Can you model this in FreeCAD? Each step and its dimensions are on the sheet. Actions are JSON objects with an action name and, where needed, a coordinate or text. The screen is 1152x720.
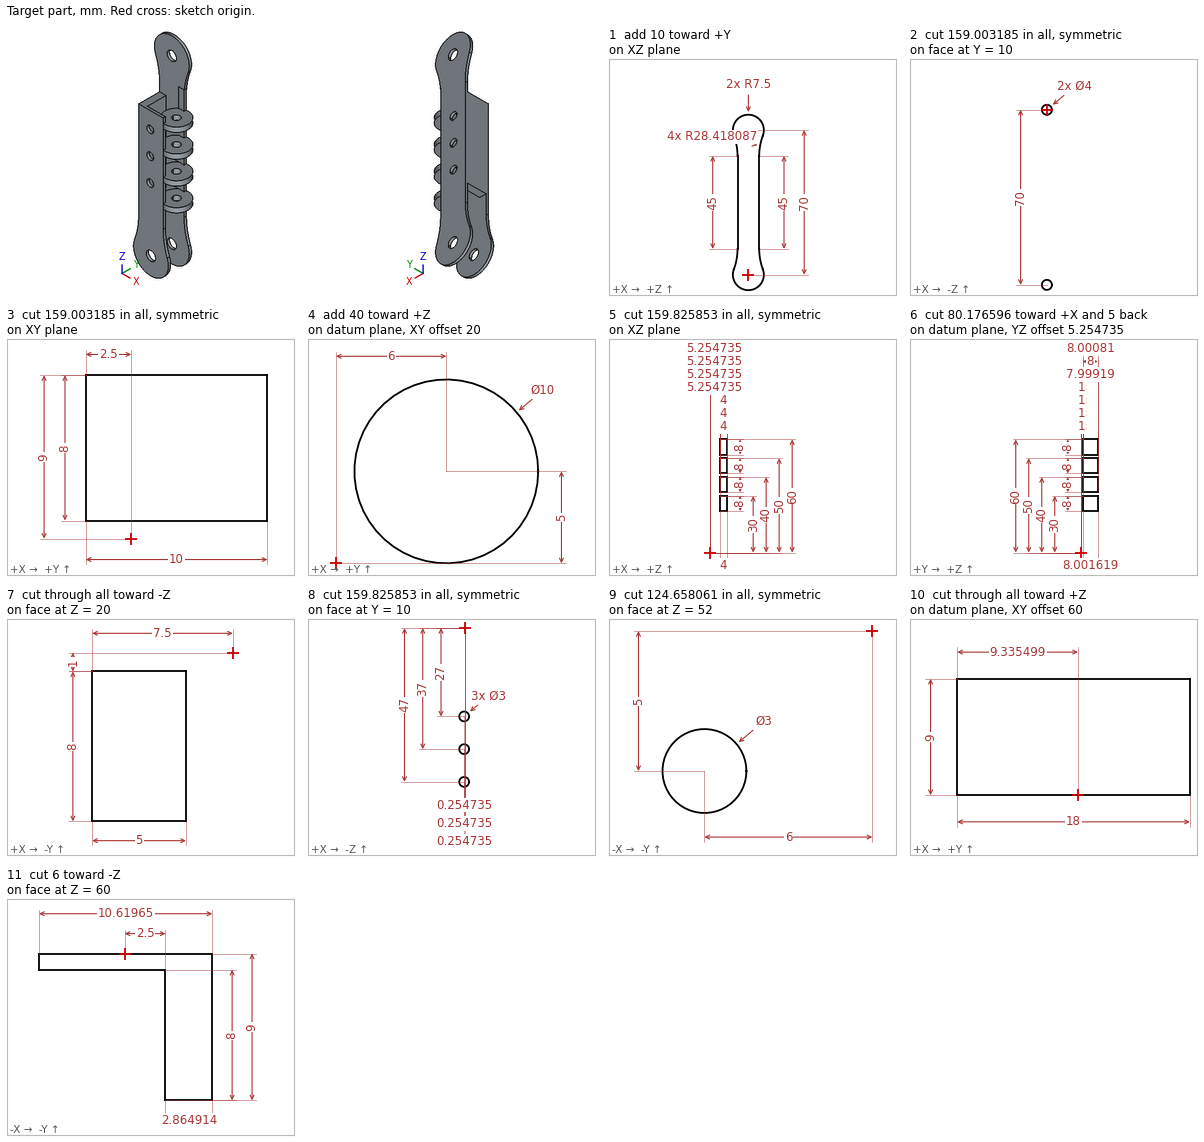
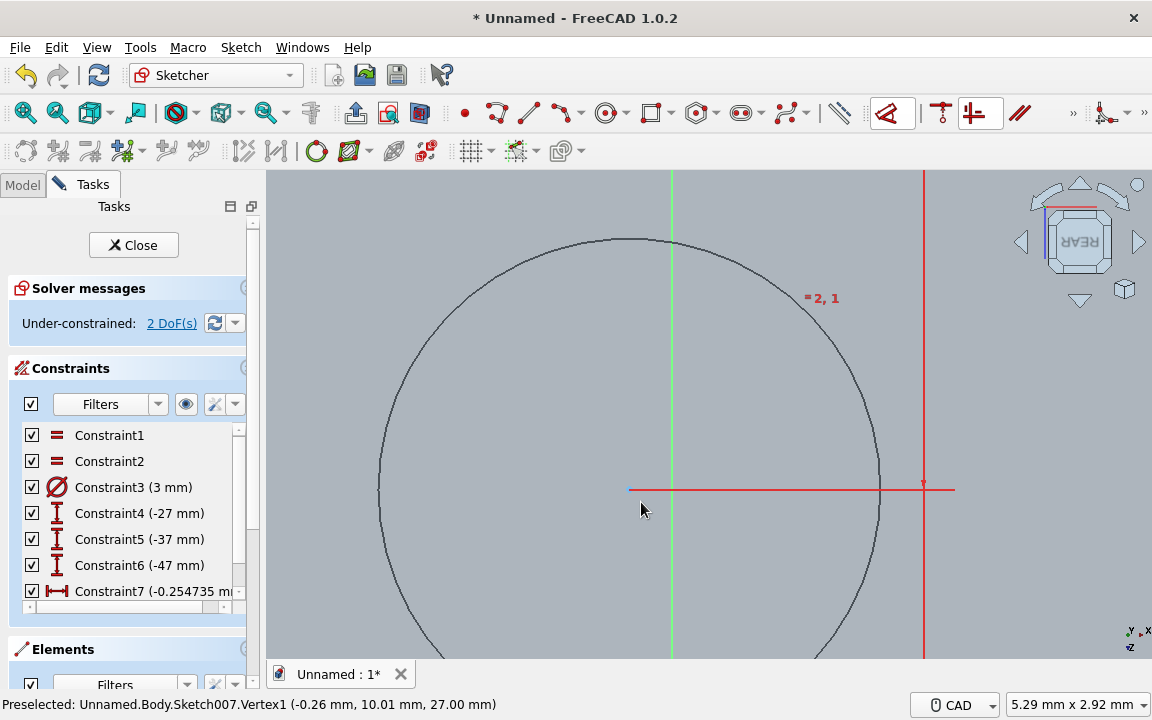
{"action": "left_click", "coordinate": [629, 490]}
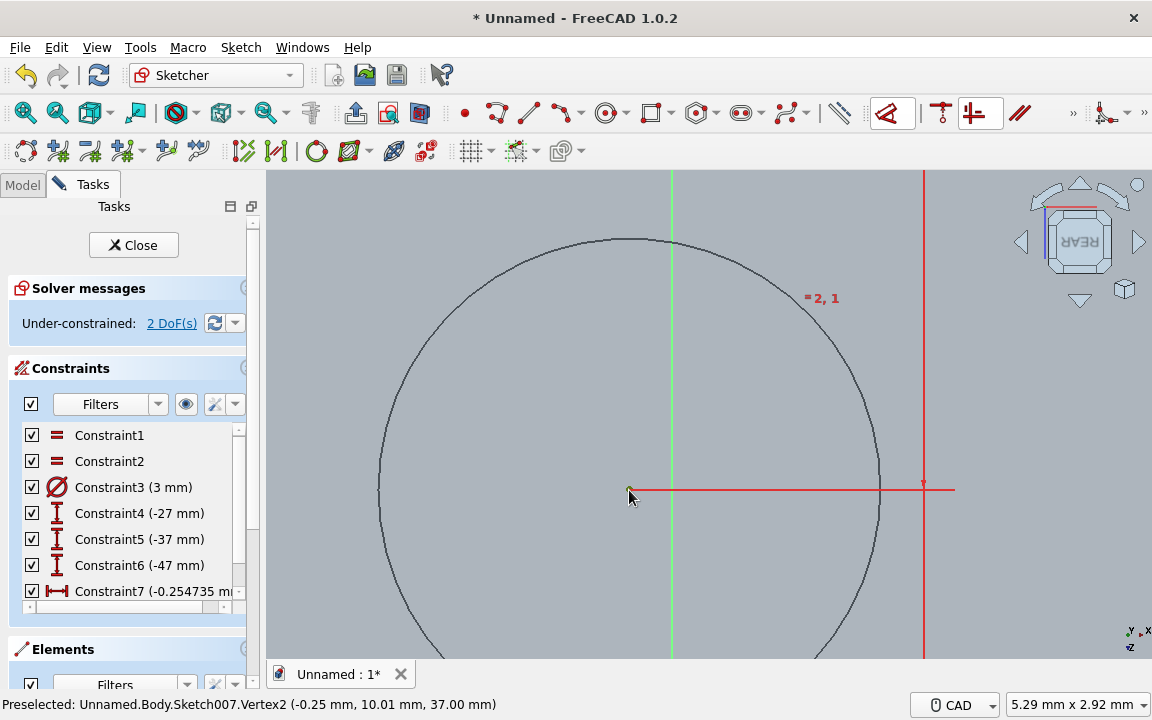
{"action": "left_click", "coordinate": [910, 114]}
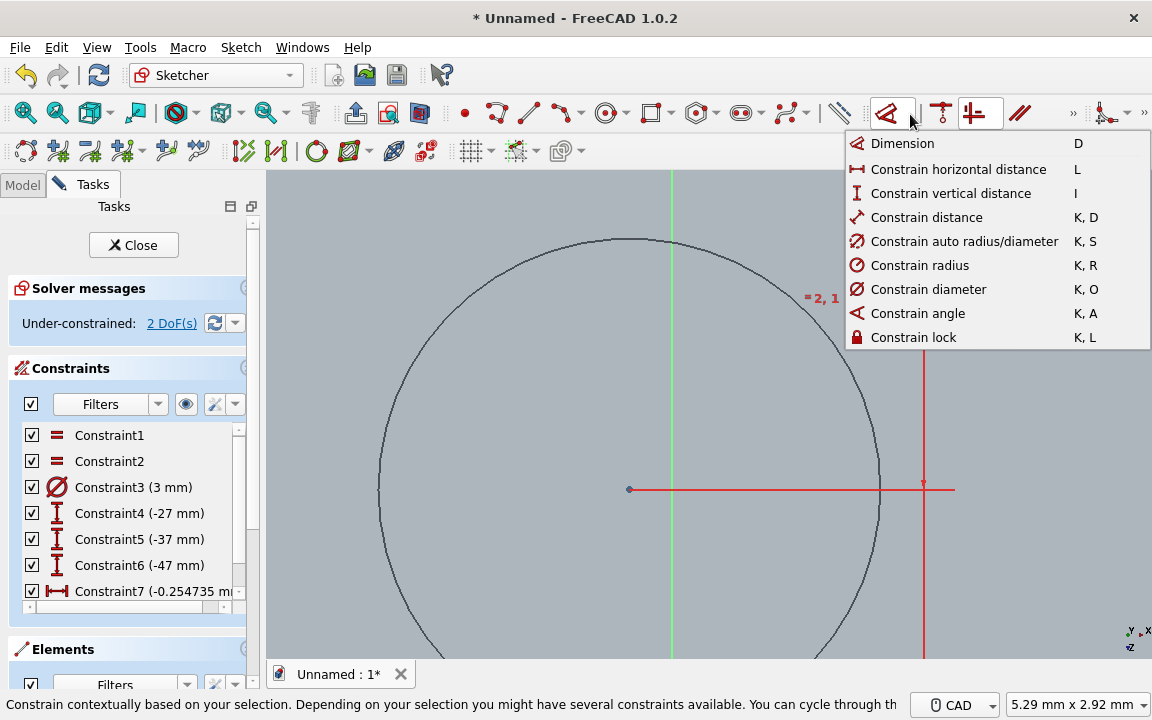
{"action": "left_click", "coordinate": [998, 169]}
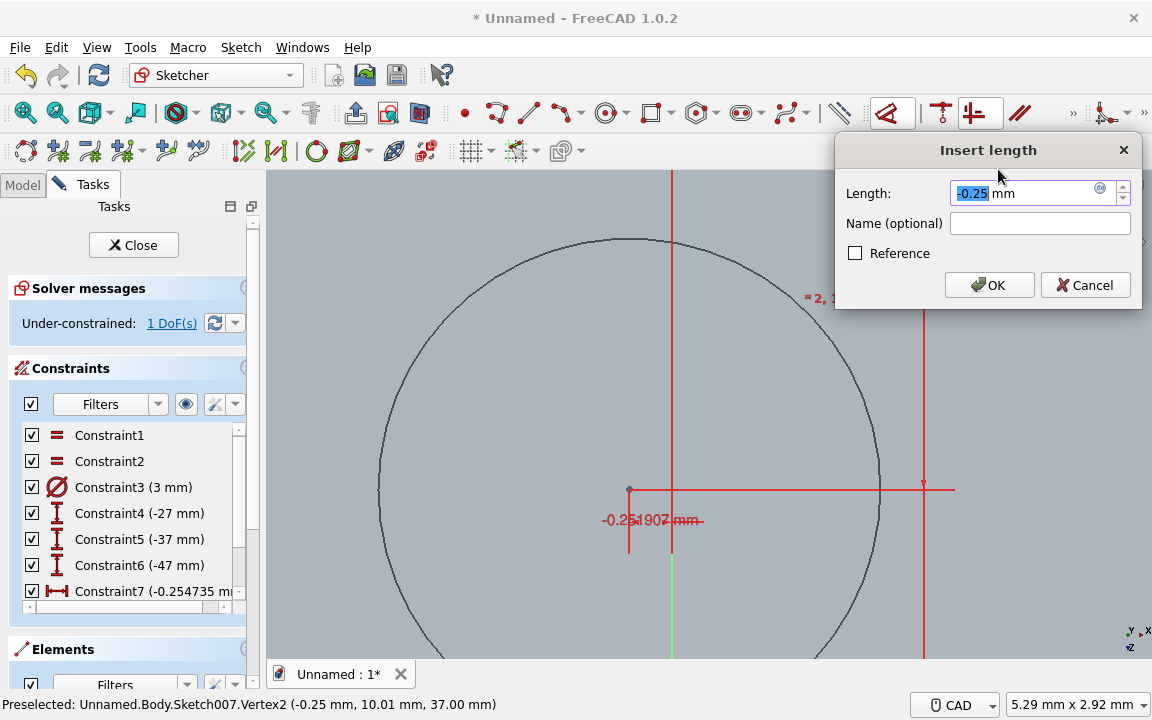
{"action": "type", "text": "-0.254735"}
{"action": "key", "text": "Return"}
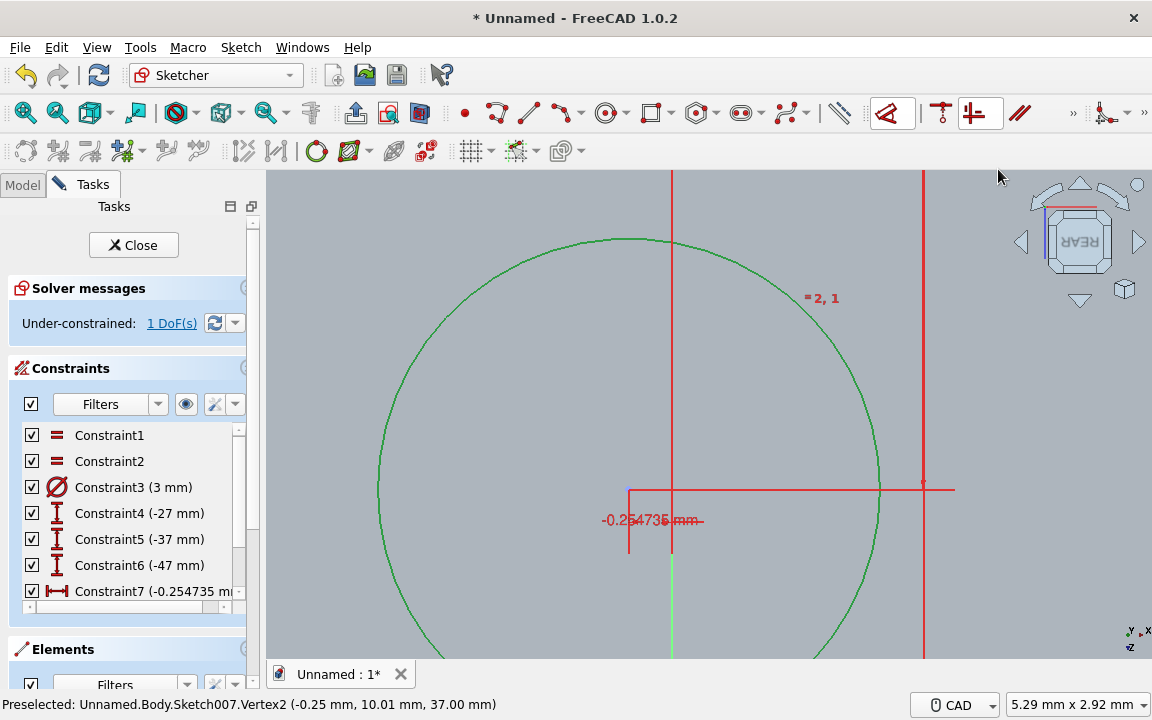
{"action": "scroll", "coordinate": [641, 502], "scroll_direction": "down", "scroll_amount": 16}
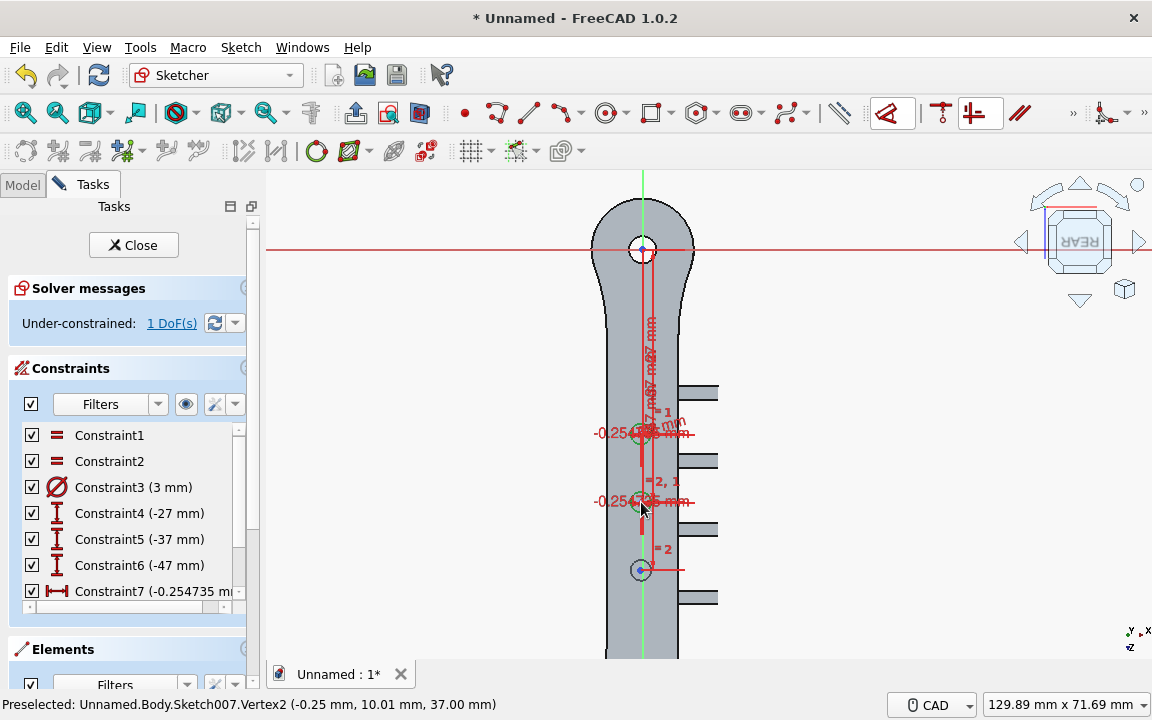
{"action": "scroll", "coordinate": [641, 570], "scroll_direction": "up", "scroll_amount": 16}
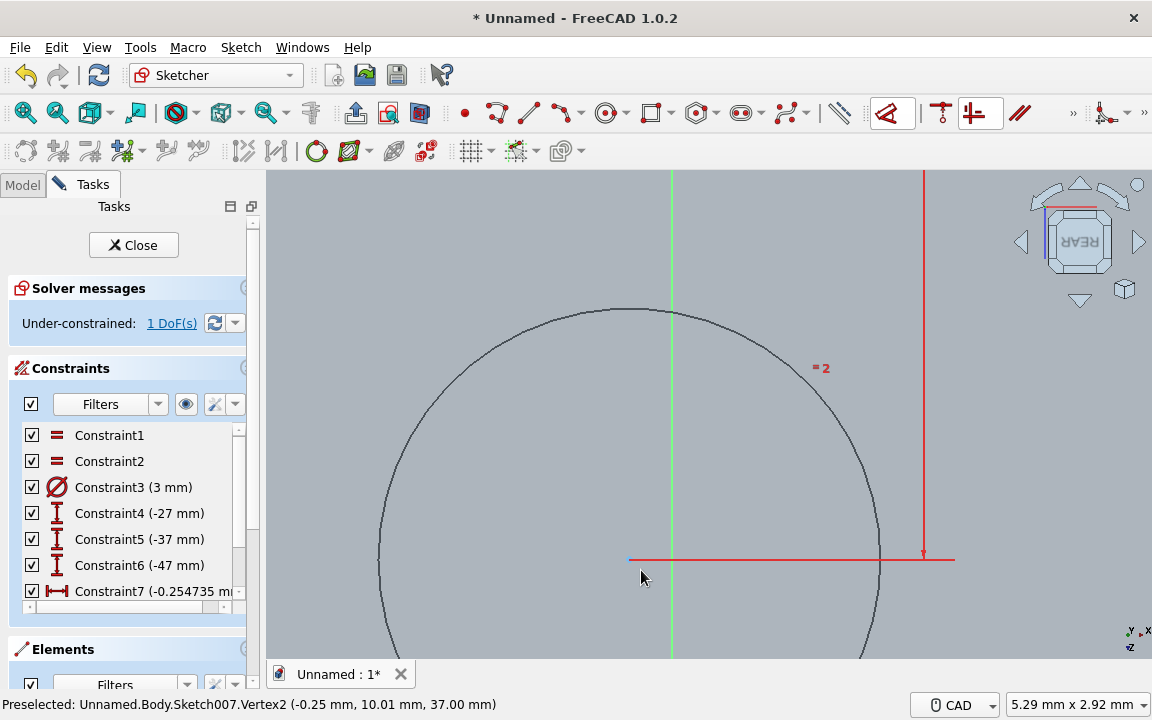
{"action": "left_click", "coordinate": [629, 560]}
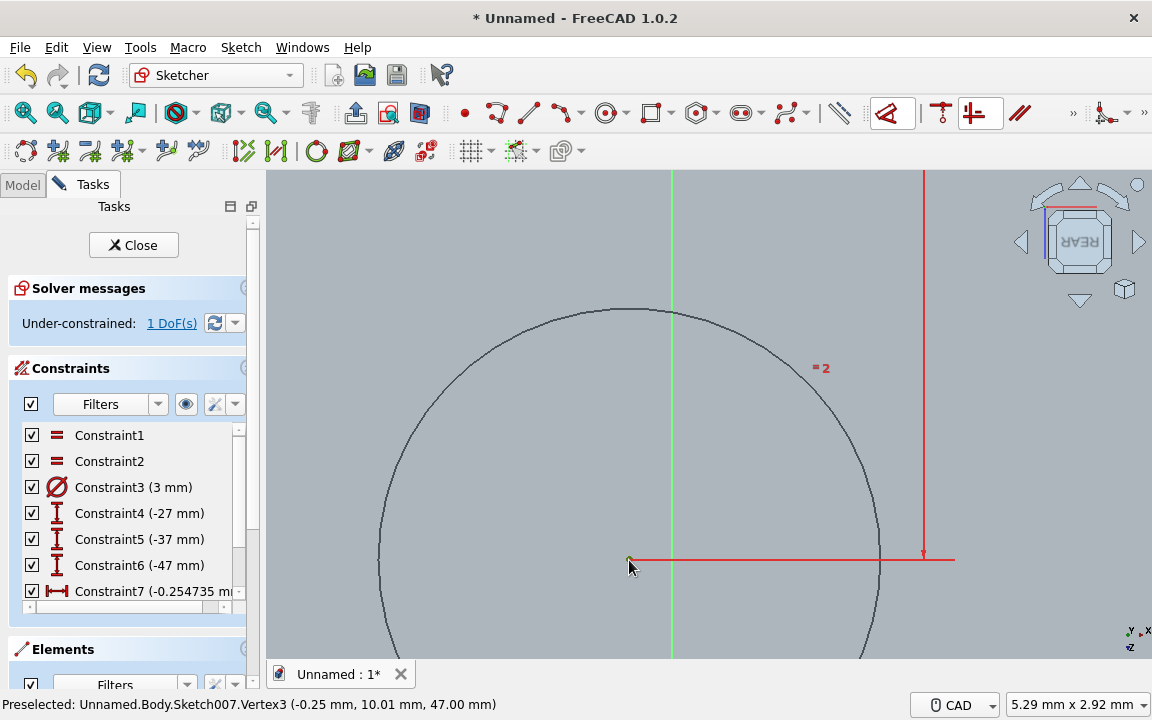
{"action": "left_click", "coordinate": [910, 114]}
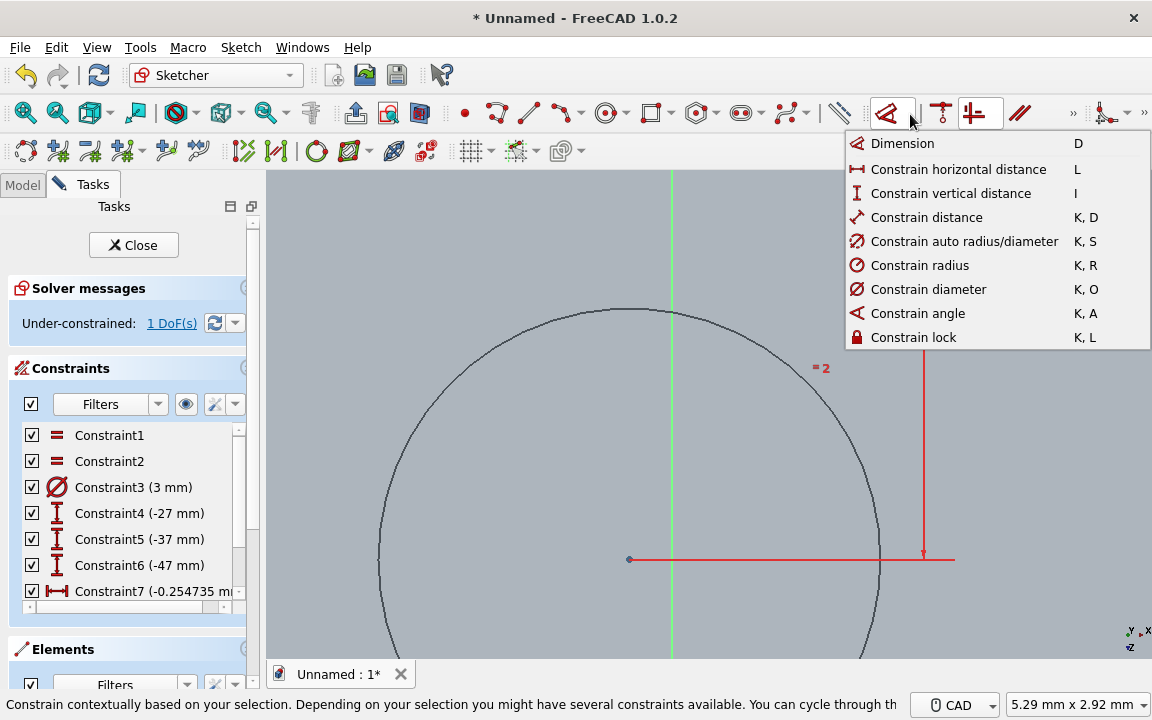
{"action": "left_click", "coordinate": [998, 169]}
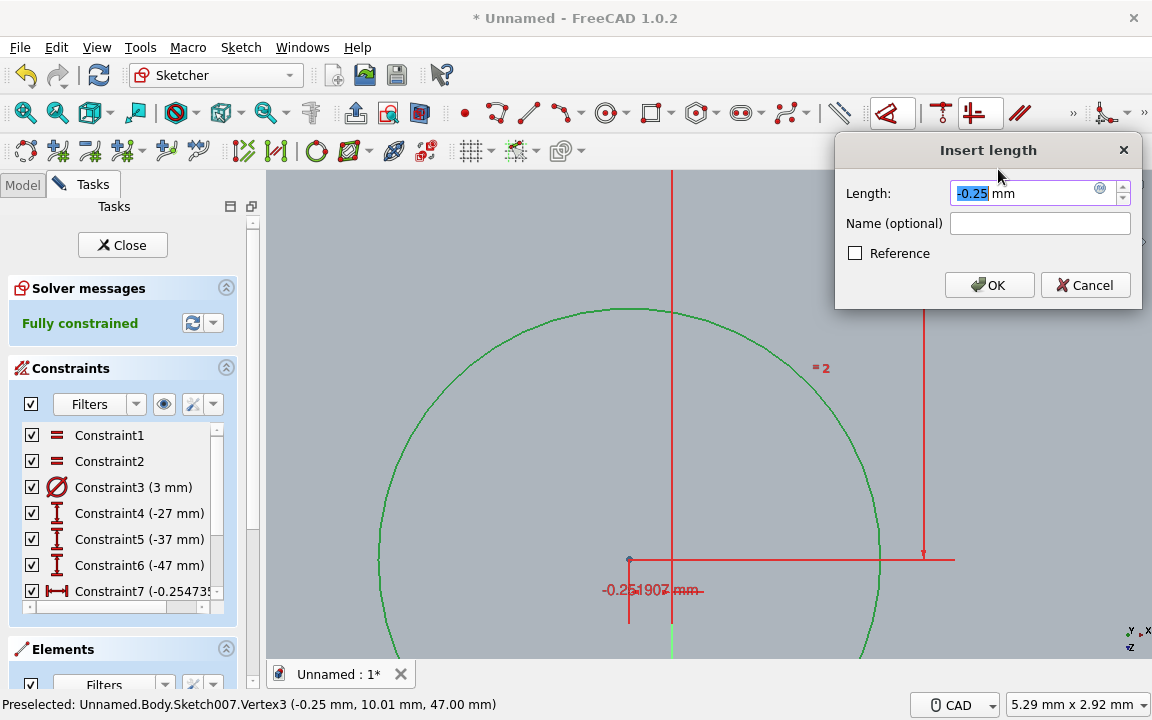
{"action": "type", "text": "-0.254735"}
{"action": "key", "text": "Return"}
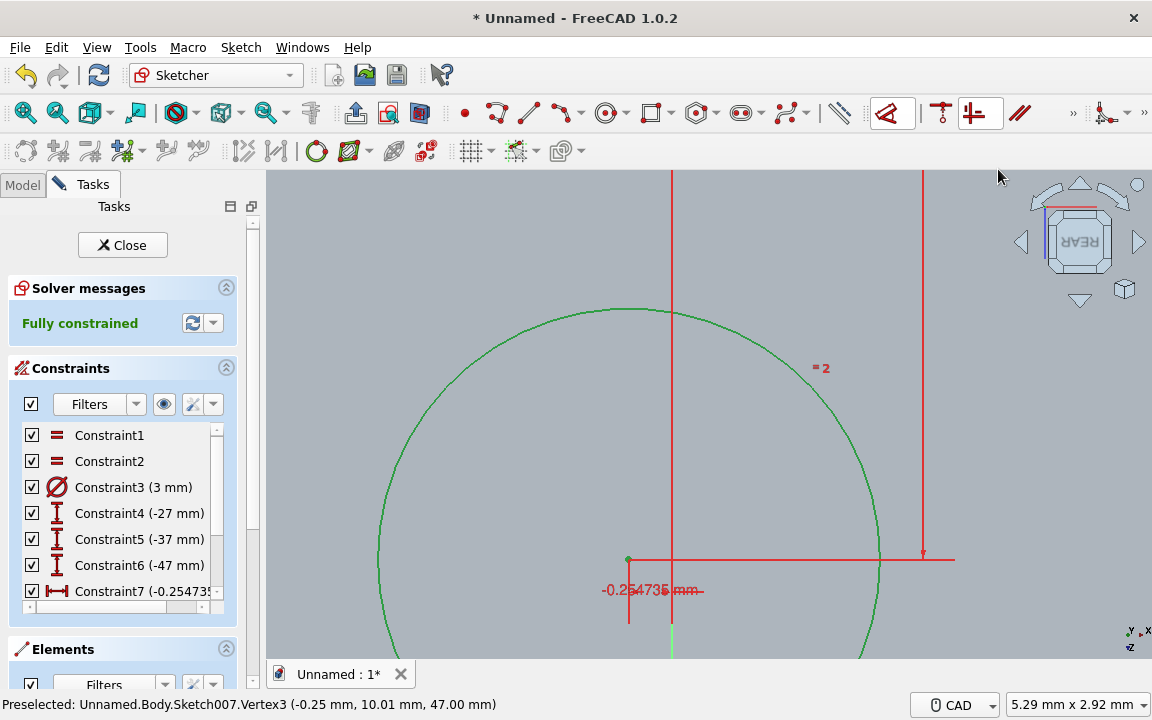
{"action": "left_click", "coordinate": [123, 245]}